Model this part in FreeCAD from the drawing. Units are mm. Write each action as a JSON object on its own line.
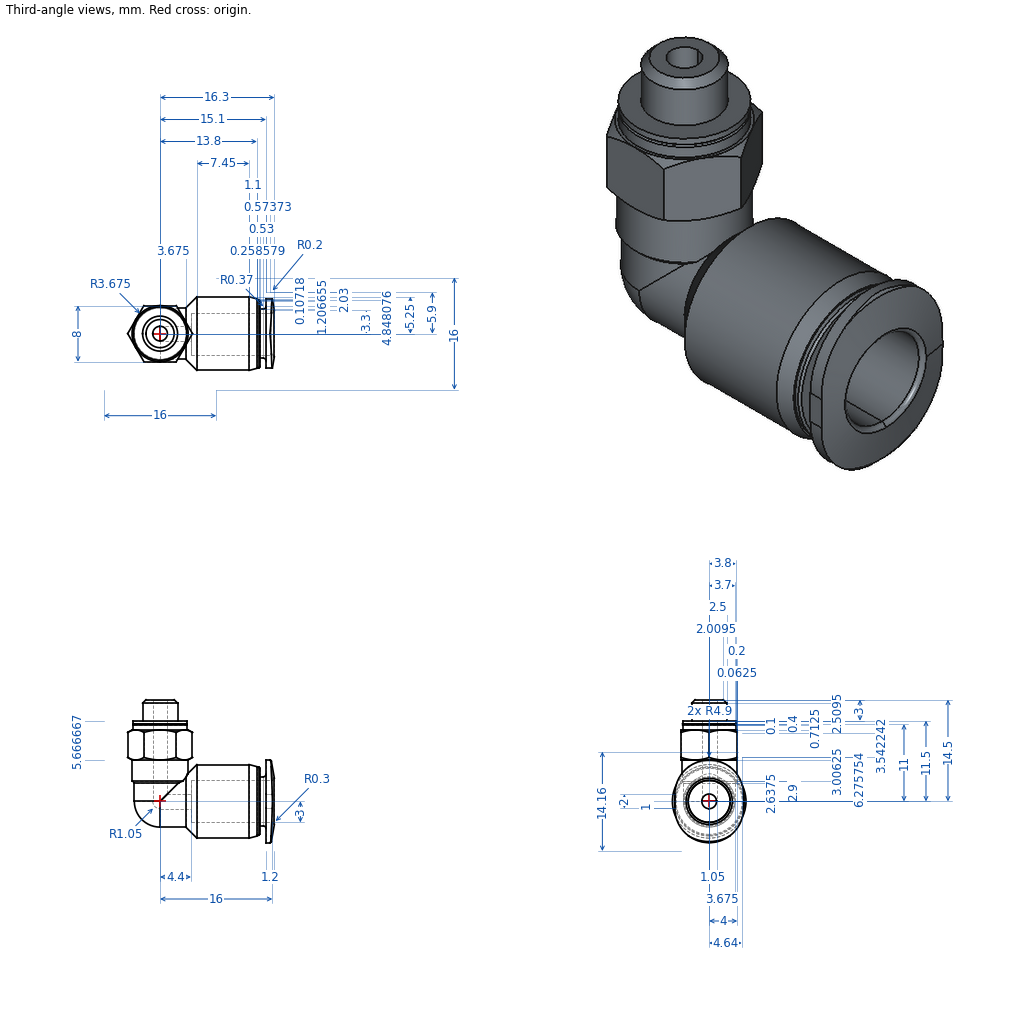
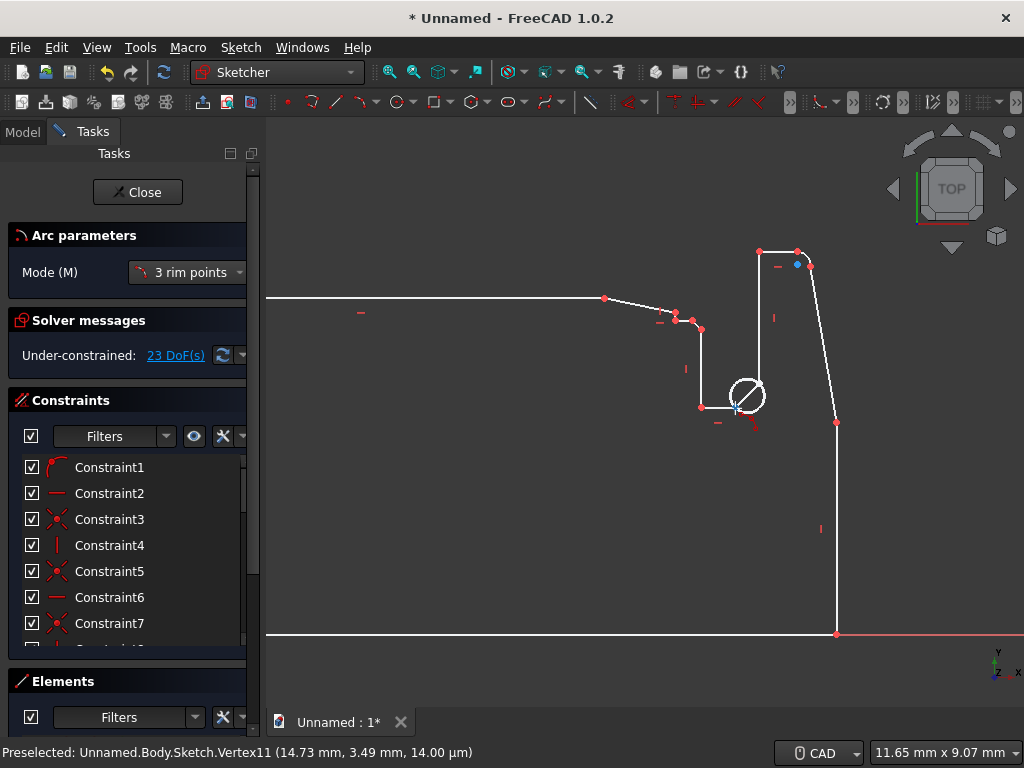
{"action": "scroll", "coordinate": [753, 400], "scroll_direction": "up", "scroll_amount": 5}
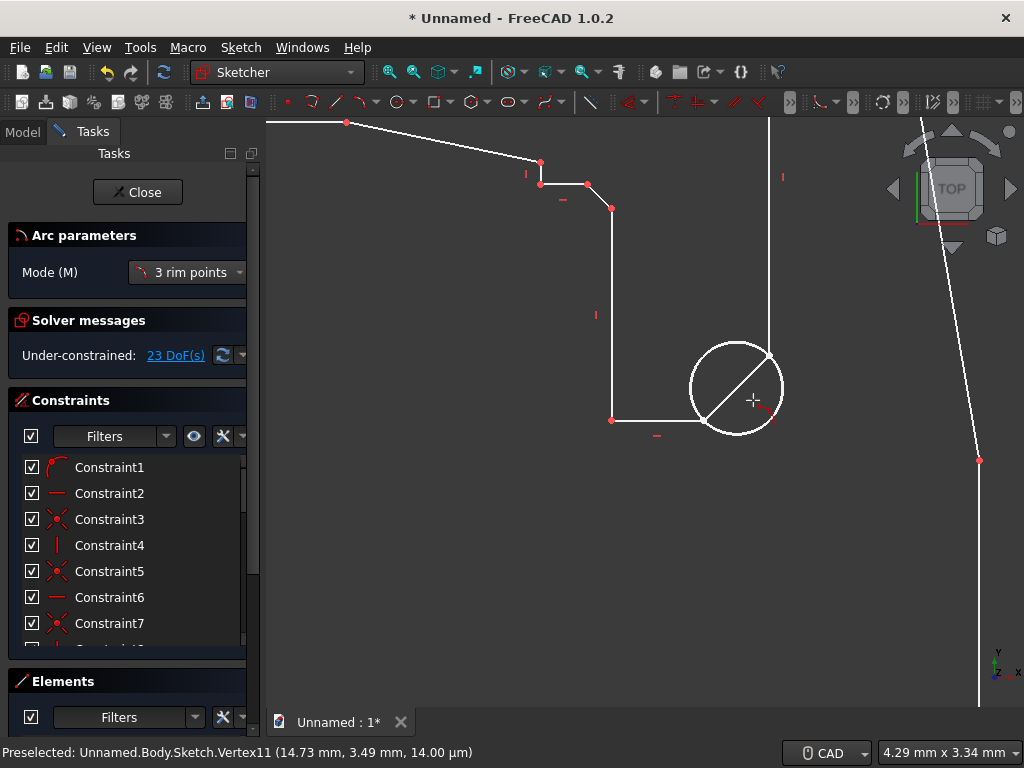
{"action": "left_click", "coordinate": [751, 400]}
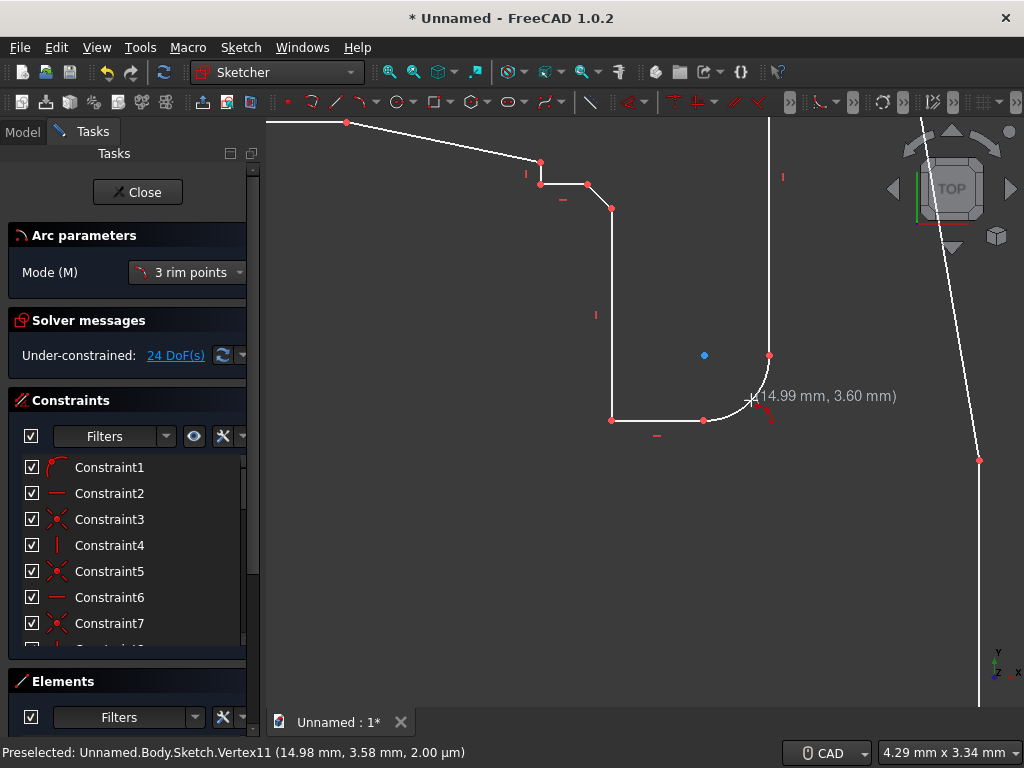
{"action": "scroll", "coordinate": [746, 399], "scroll_direction": "down", "scroll_amount": 11}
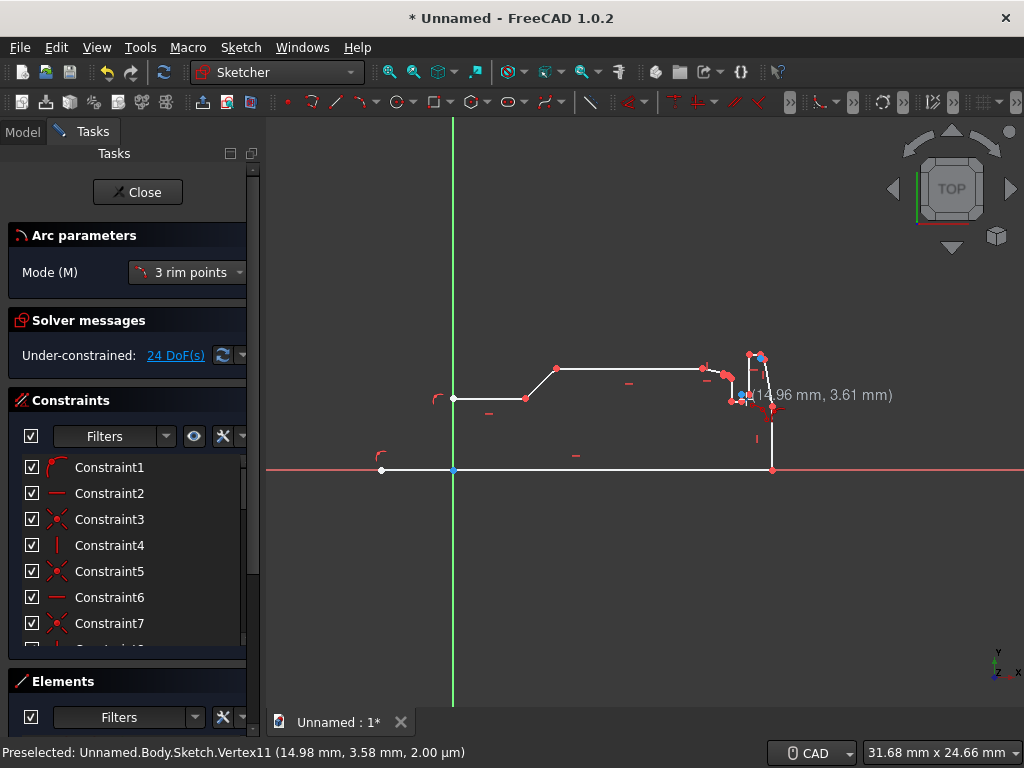
{"action": "left_click", "coordinate": [453, 399]}
{"action": "left_click", "coordinate": [381, 470]}
{"action": "left_click", "coordinate": [403, 419]}
{"action": "key", "text": "Escape"}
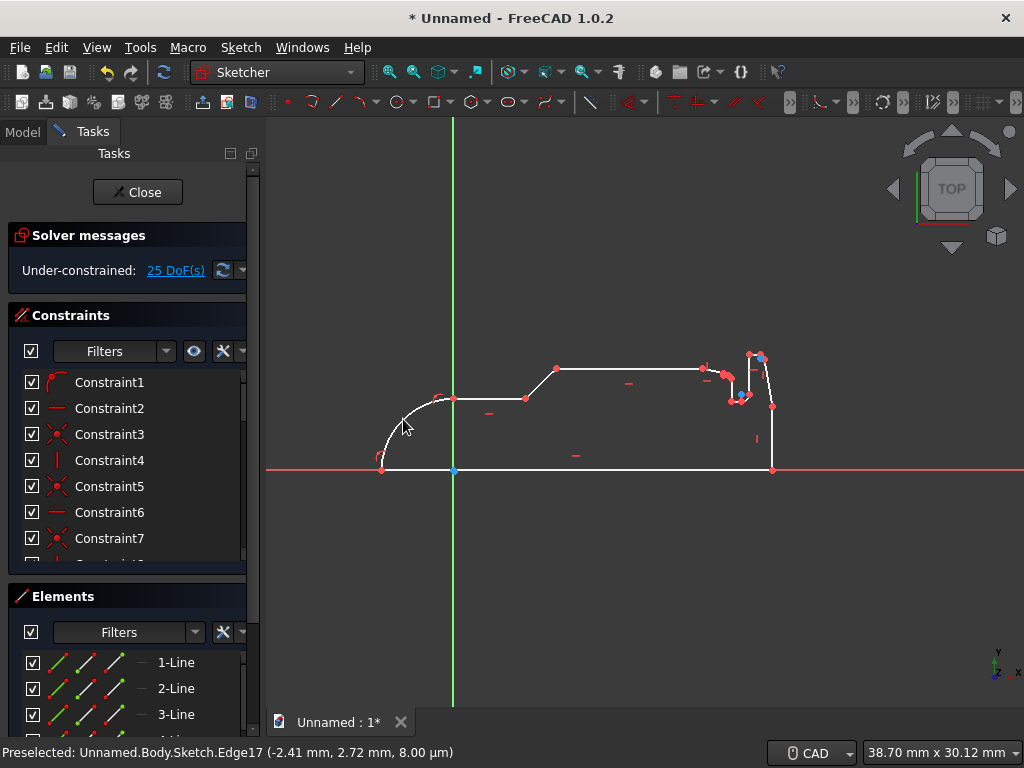
{"action": "left_click", "coordinate": [770, 392]}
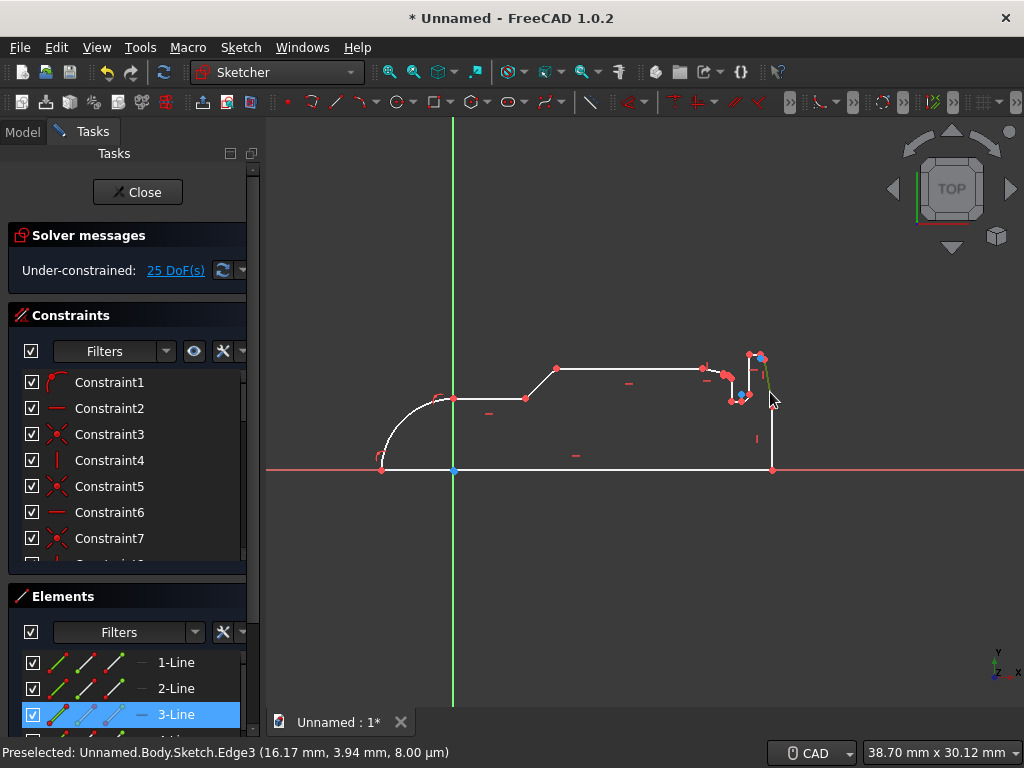
{"action": "scroll", "coordinate": [764, 356], "scroll_direction": "up", "scroll_amount": 8}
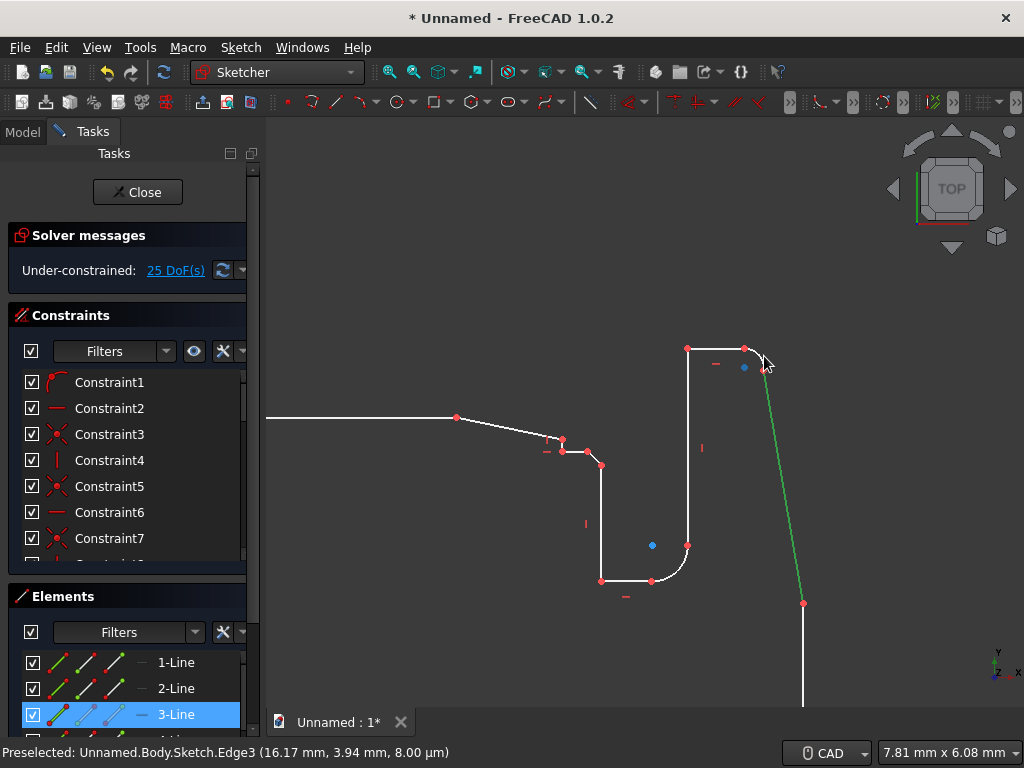
{"action": "left_click", "coordinate": [759, 355]}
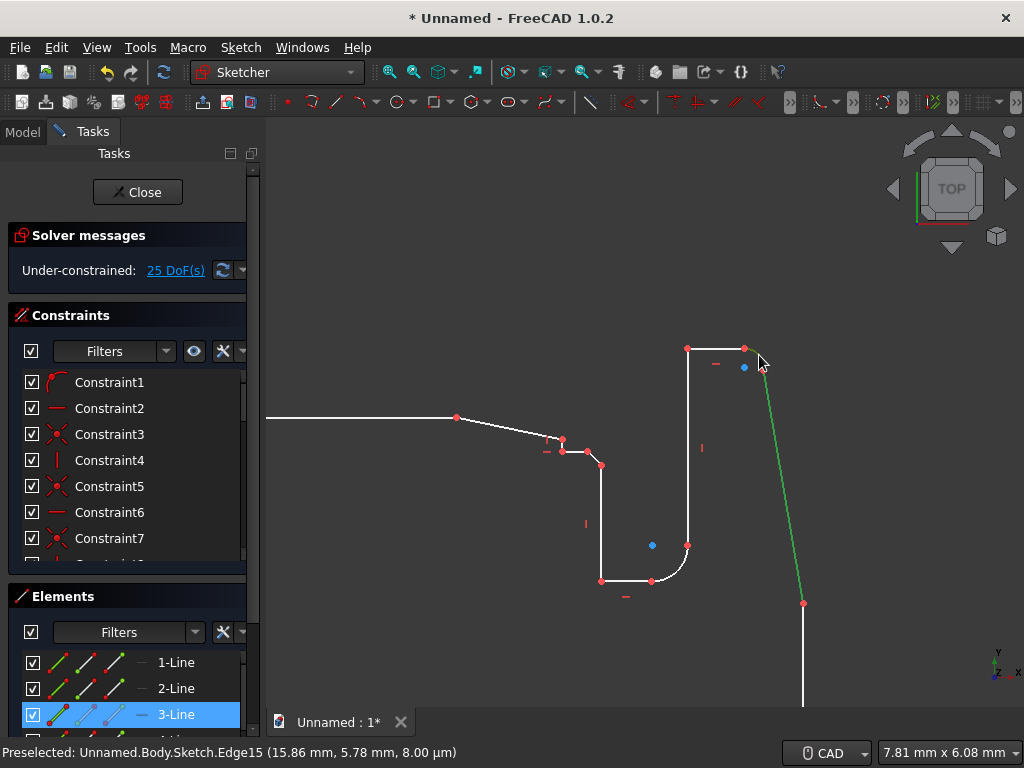
{"action": "key", "text": "t"}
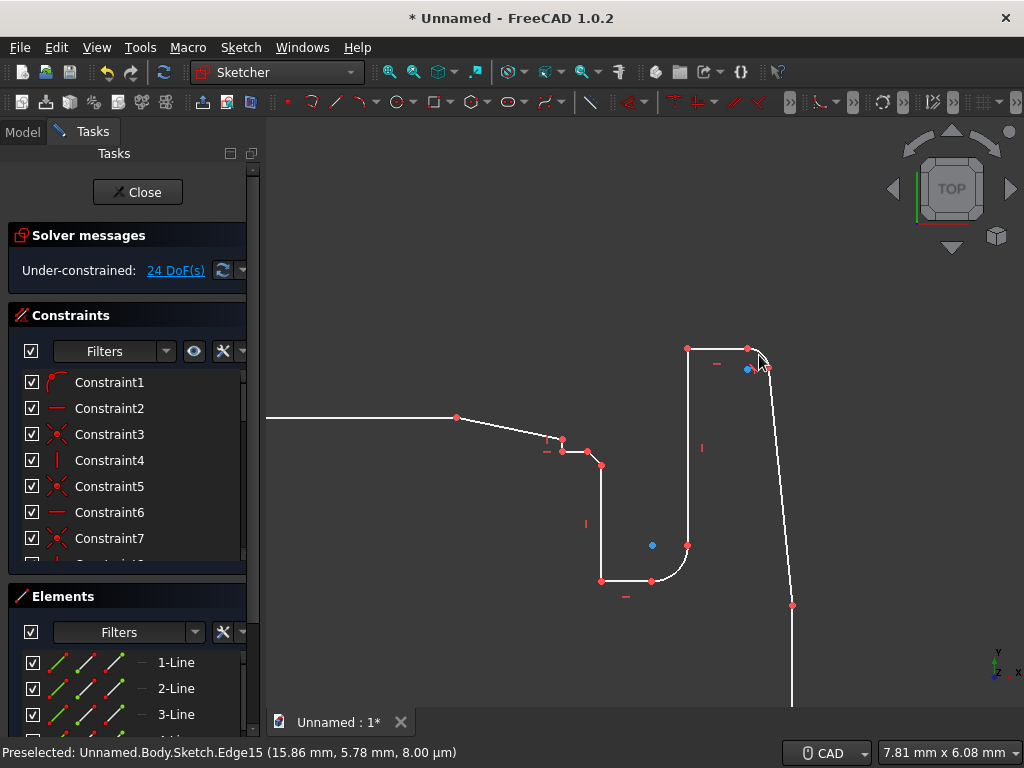
{"action": "left_click", "coordinate": [729, 349]}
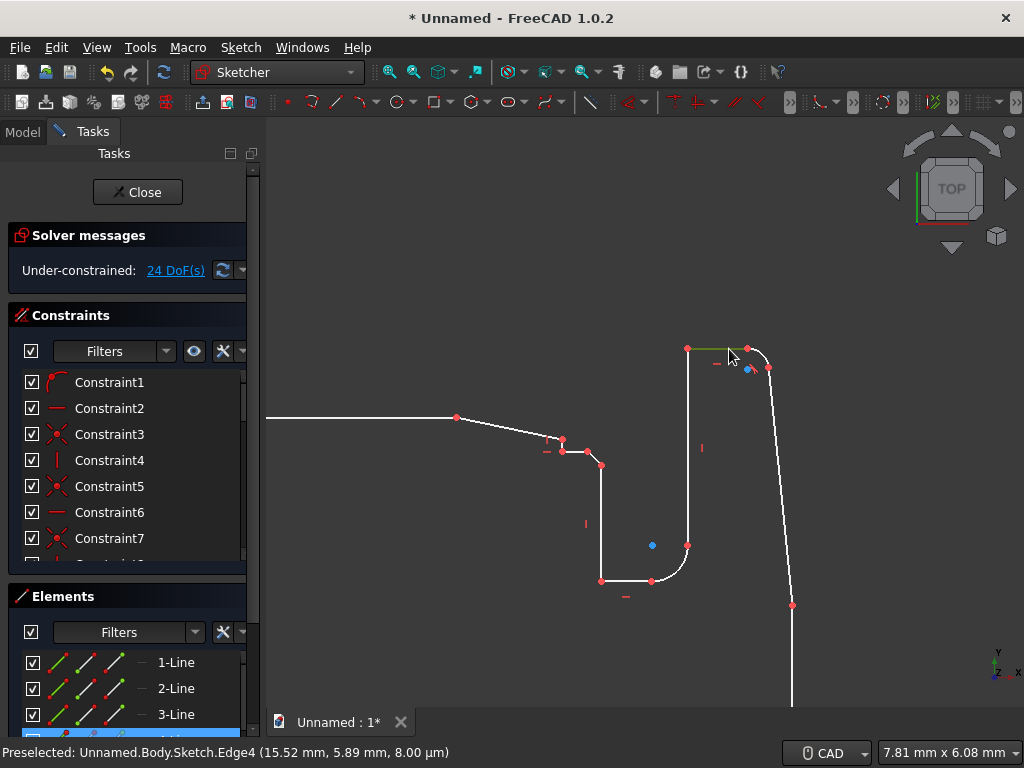
{"action": "scroll", "coordinate": [766, 358], "scroll_direction": "up", "scroll_amount": 2}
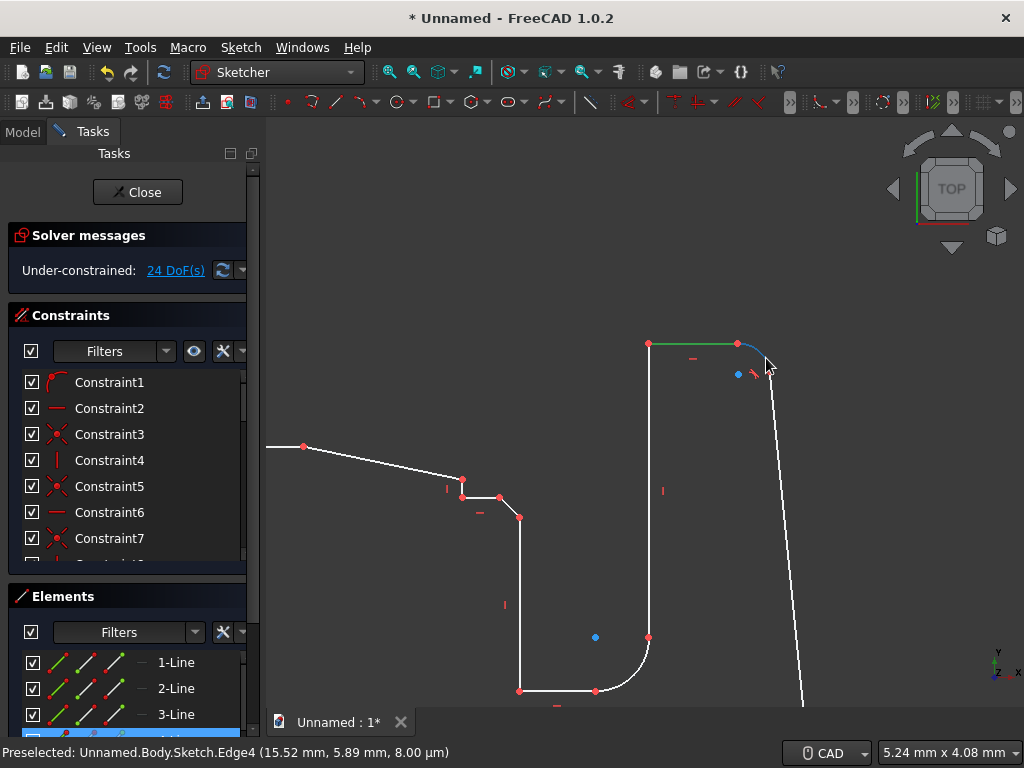
{"action": "left_click", "coordinate": [765, 359]}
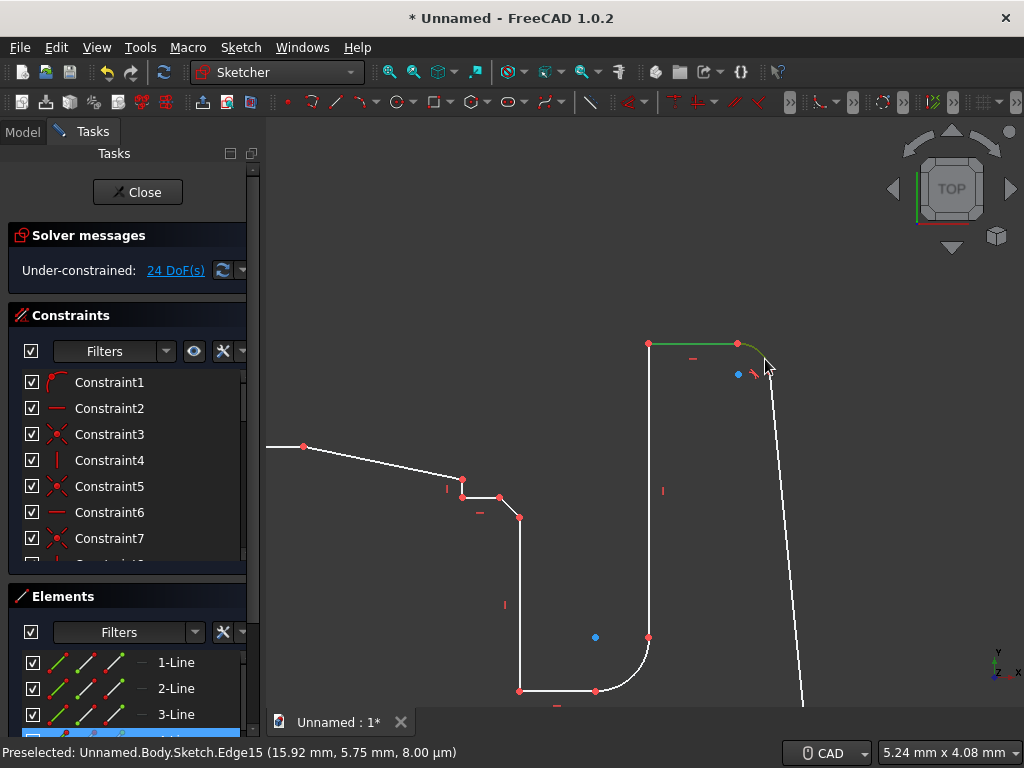
{"action": "key", "text": "t"}